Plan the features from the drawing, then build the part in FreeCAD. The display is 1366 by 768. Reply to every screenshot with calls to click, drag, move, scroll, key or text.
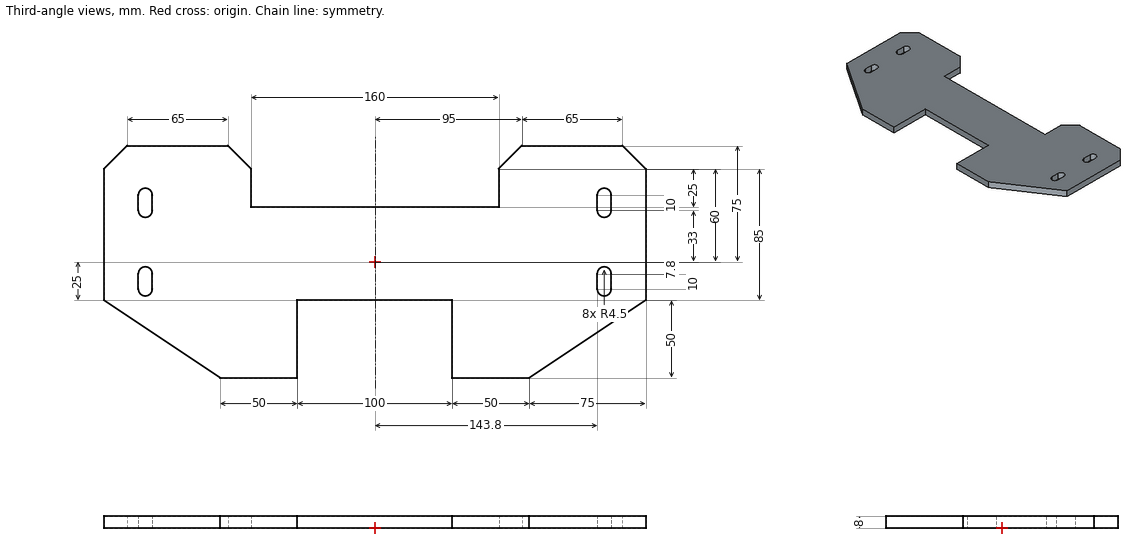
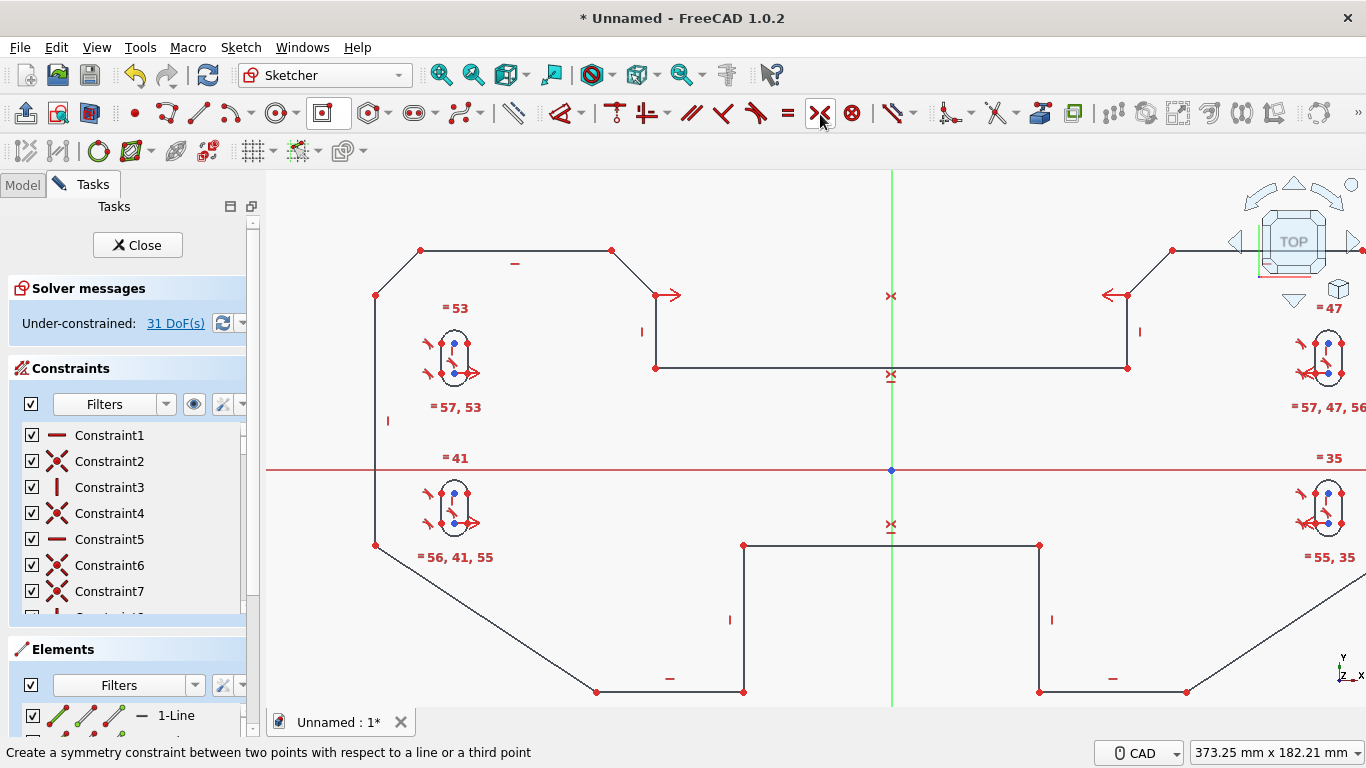
click(1172, 251)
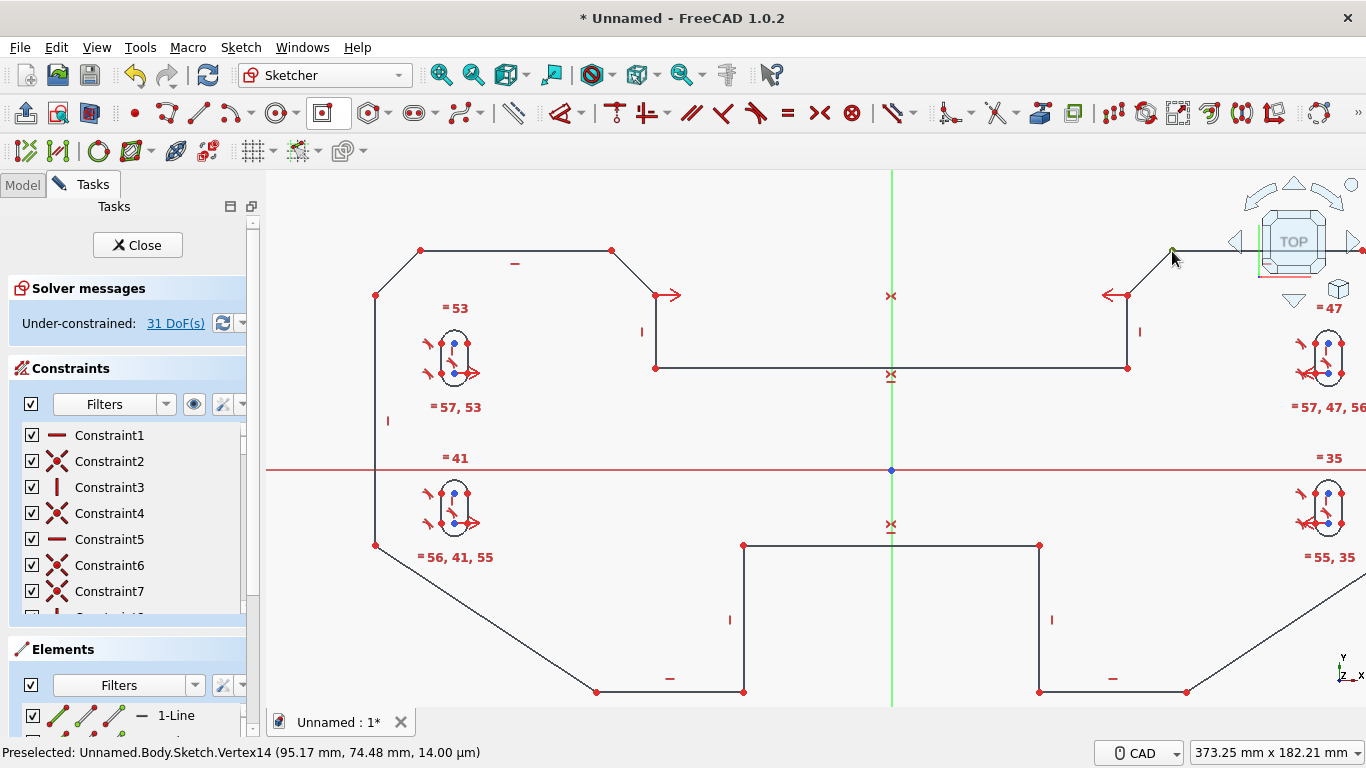
click(611, 251)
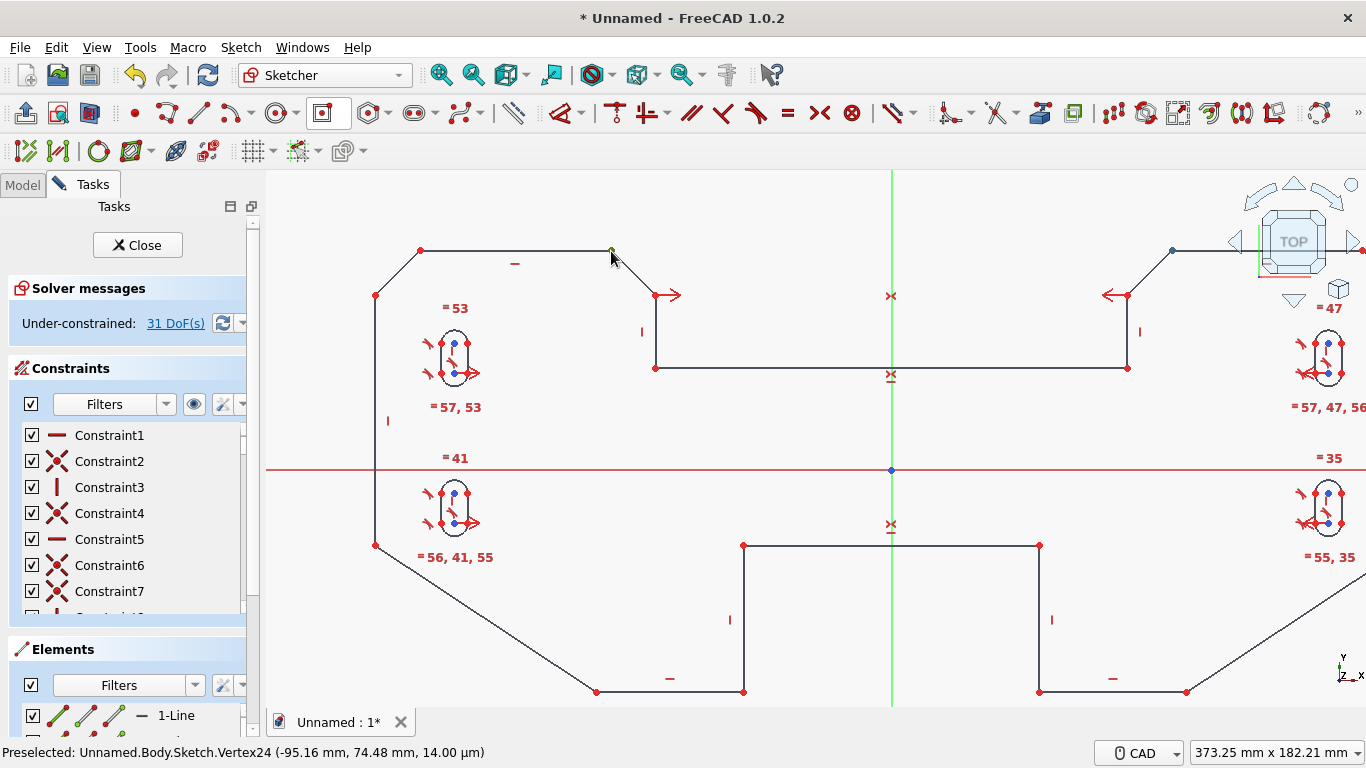
click(892, 645)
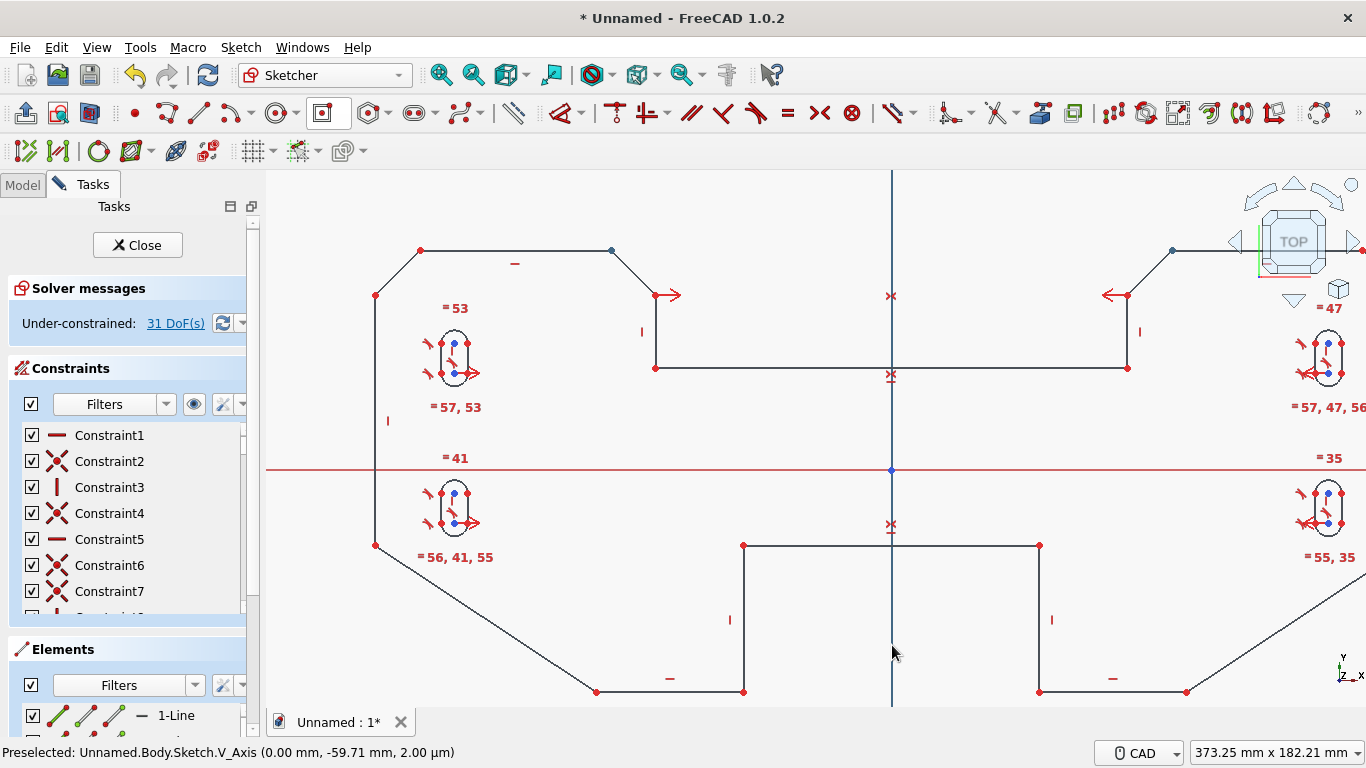
click(820, 114)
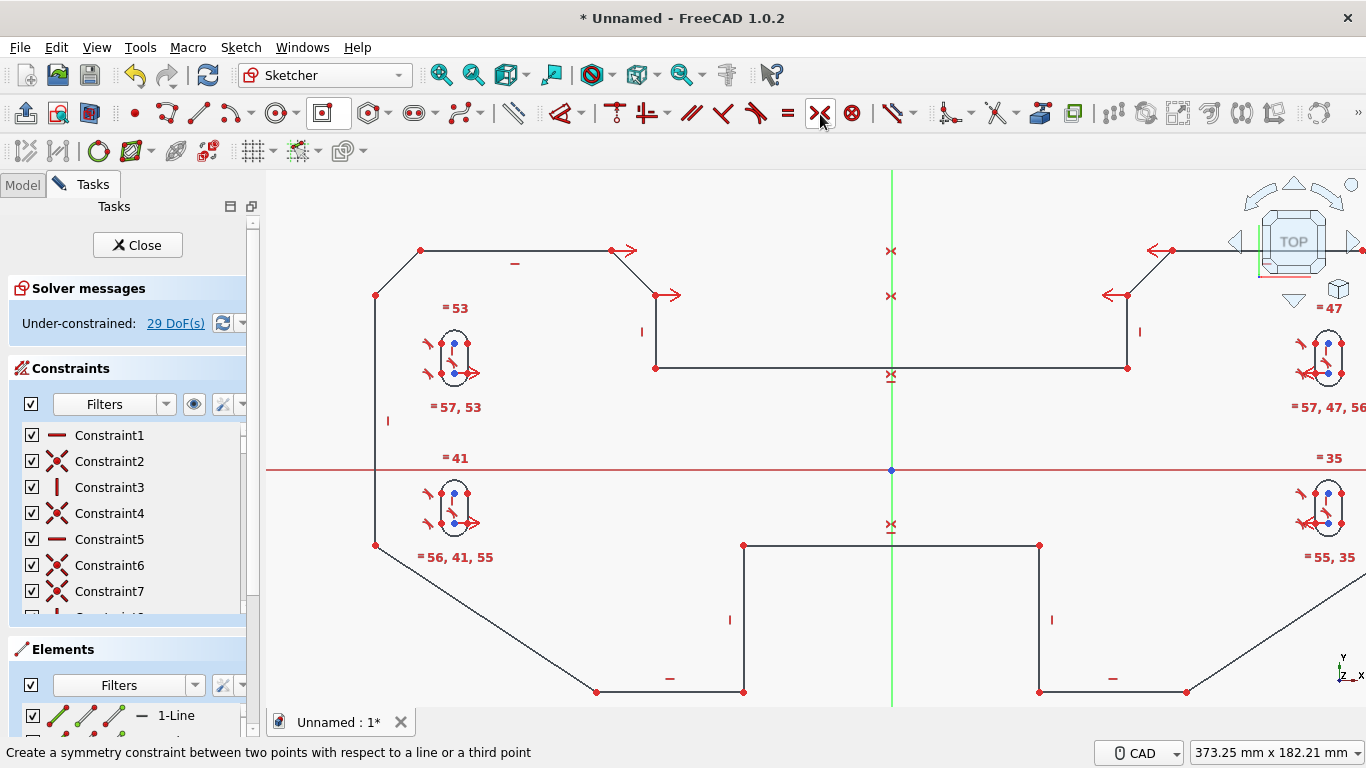
scroll(455, 374, down, 2)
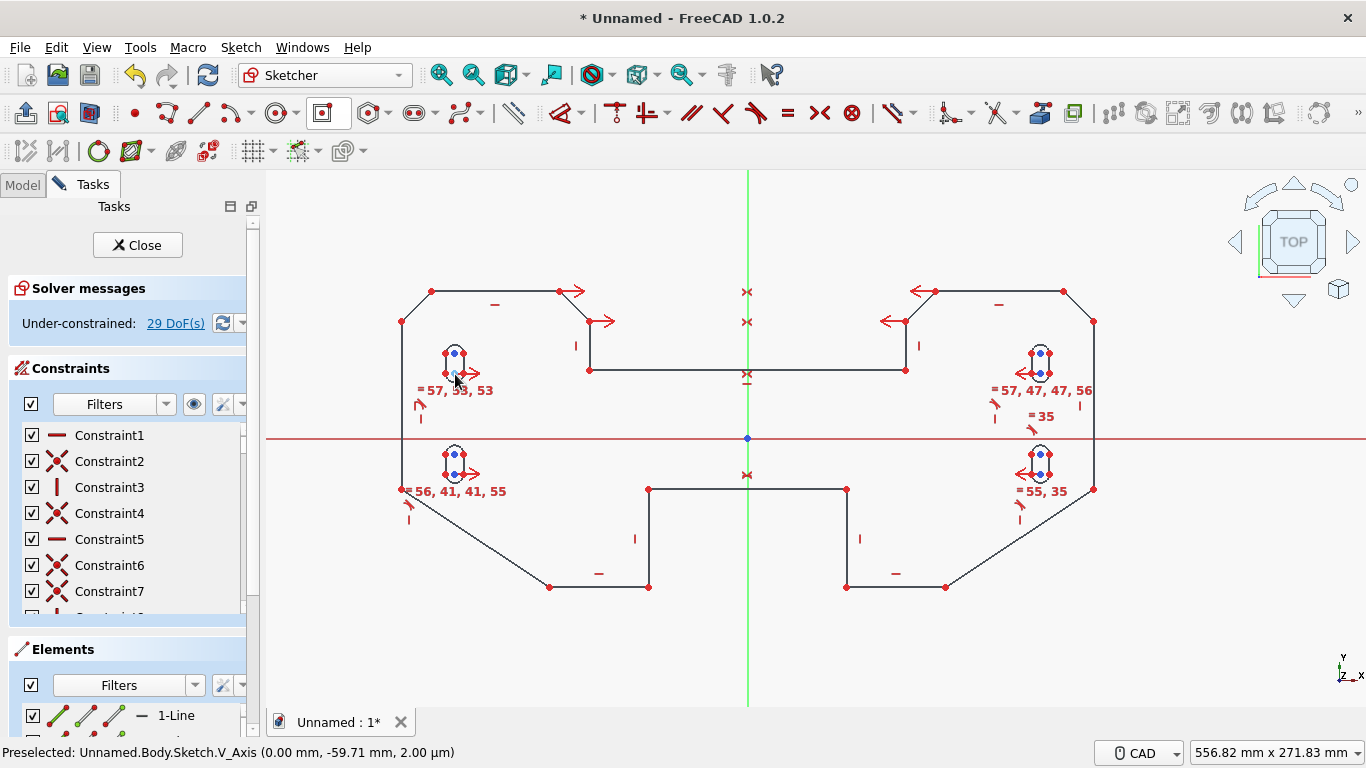
click(1094, 321)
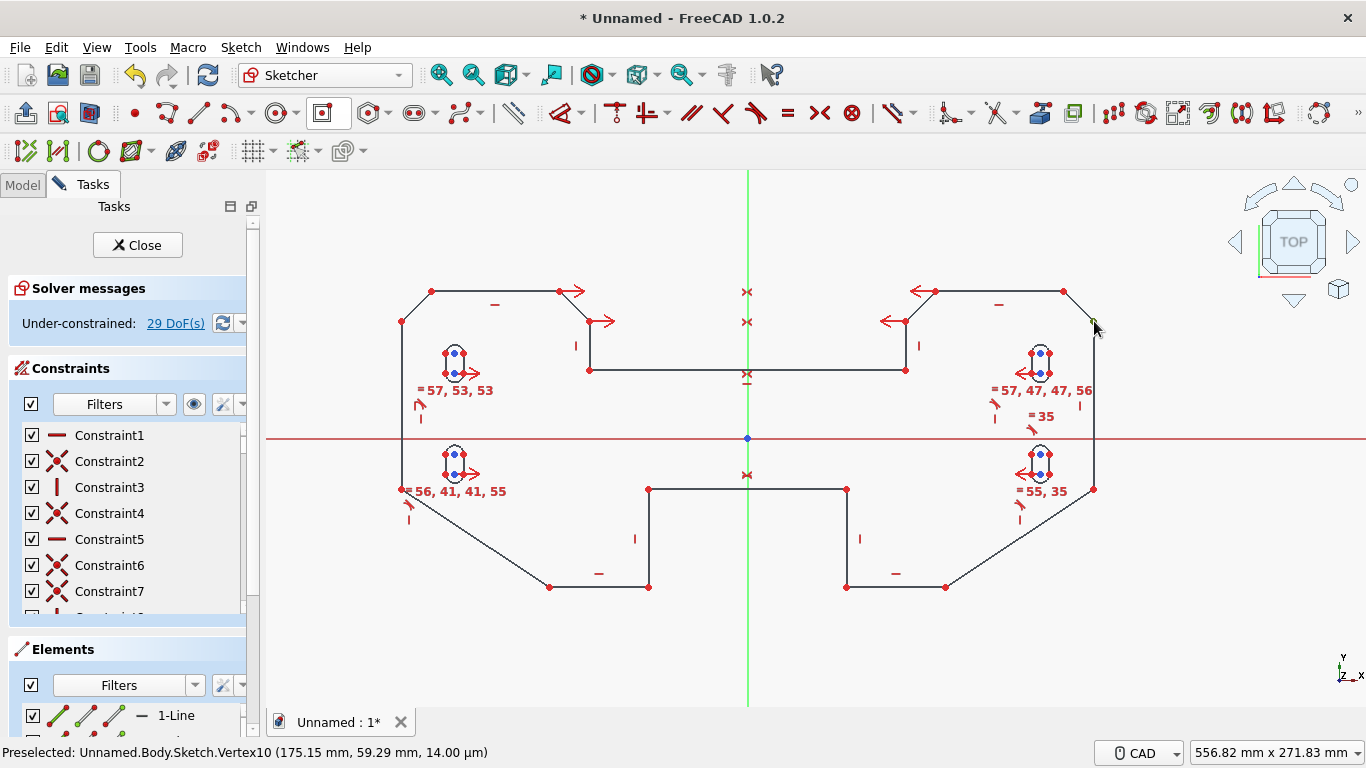
click(402, 321)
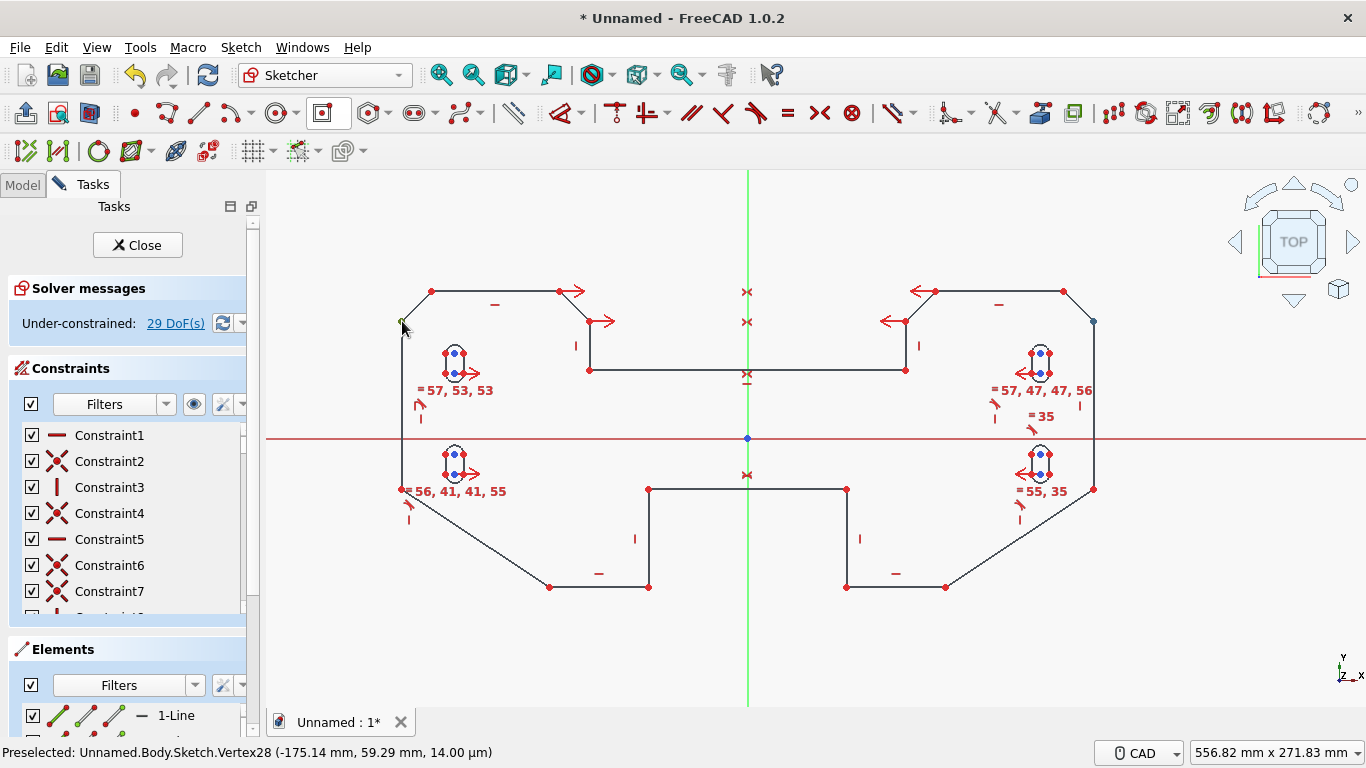
click(748, 645)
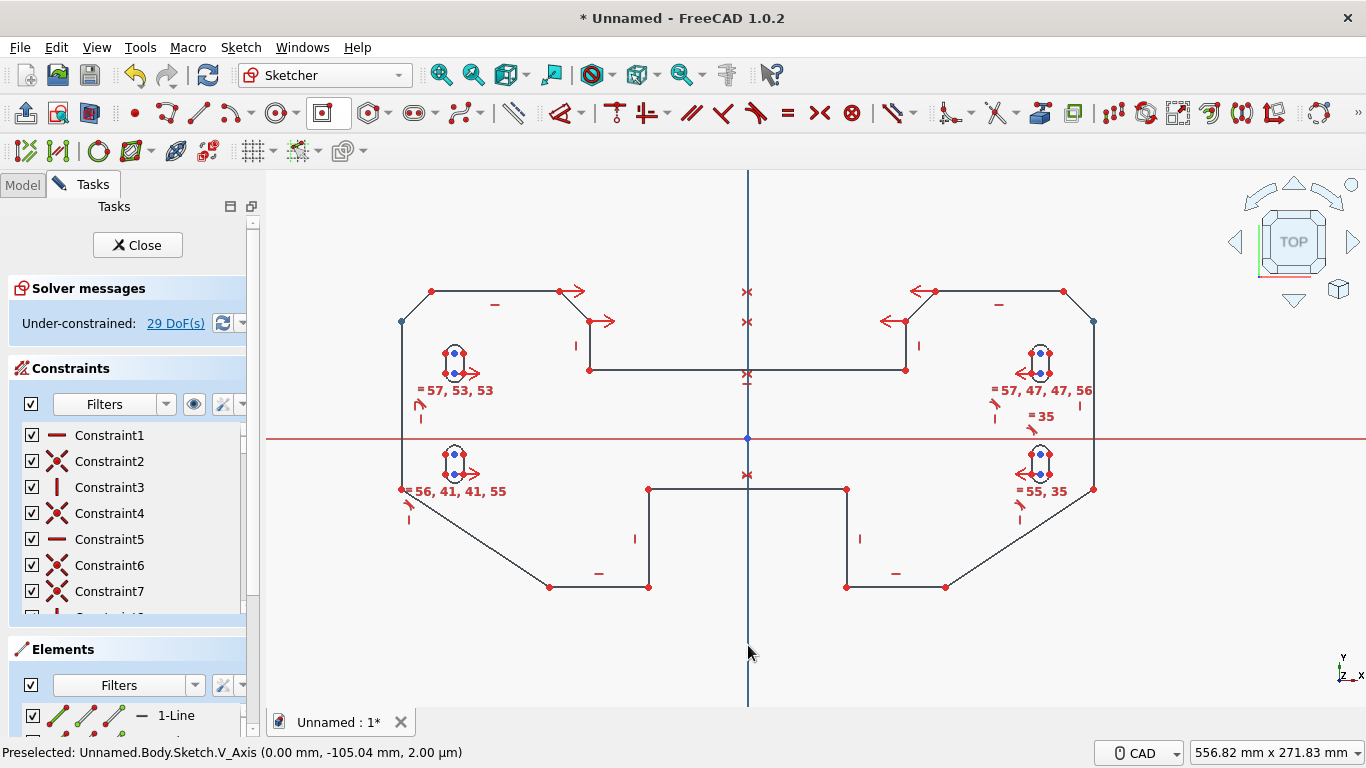
click(820, 114)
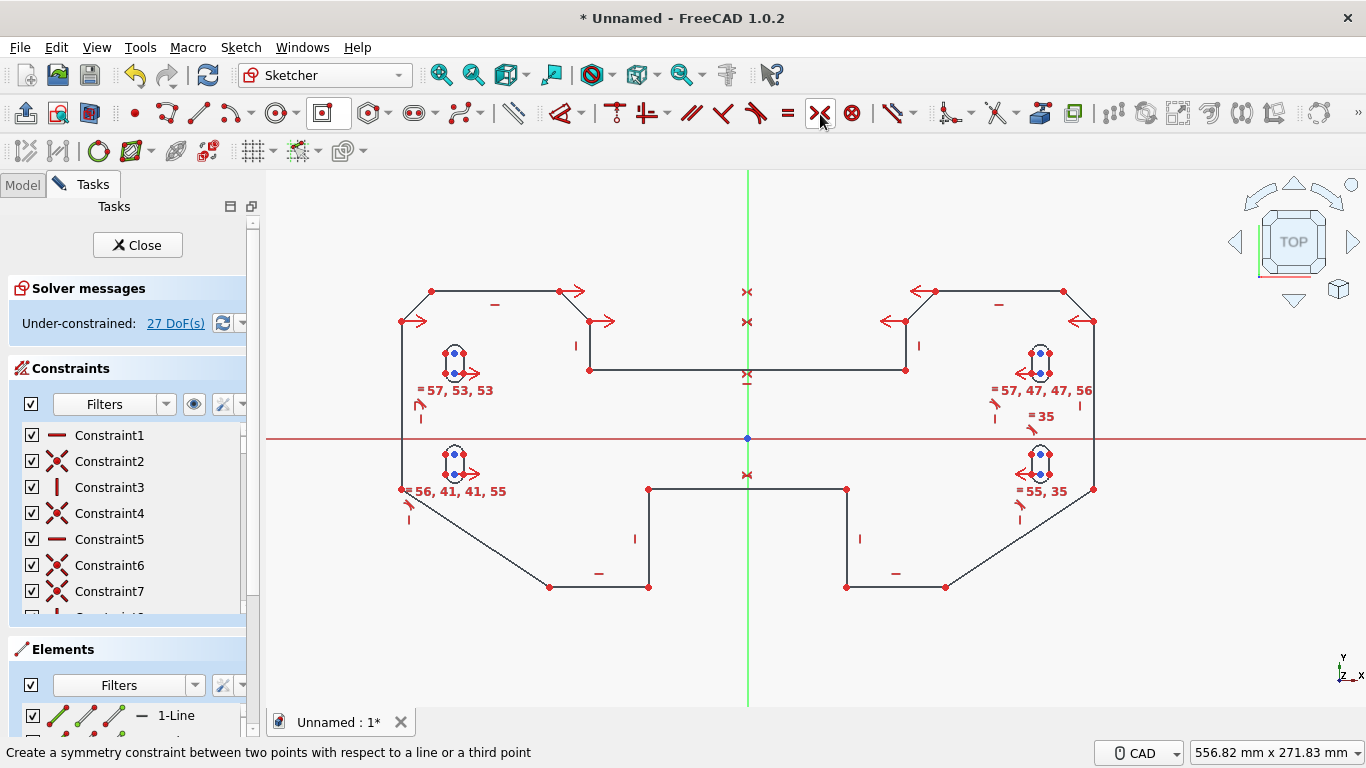
click(946, 587)